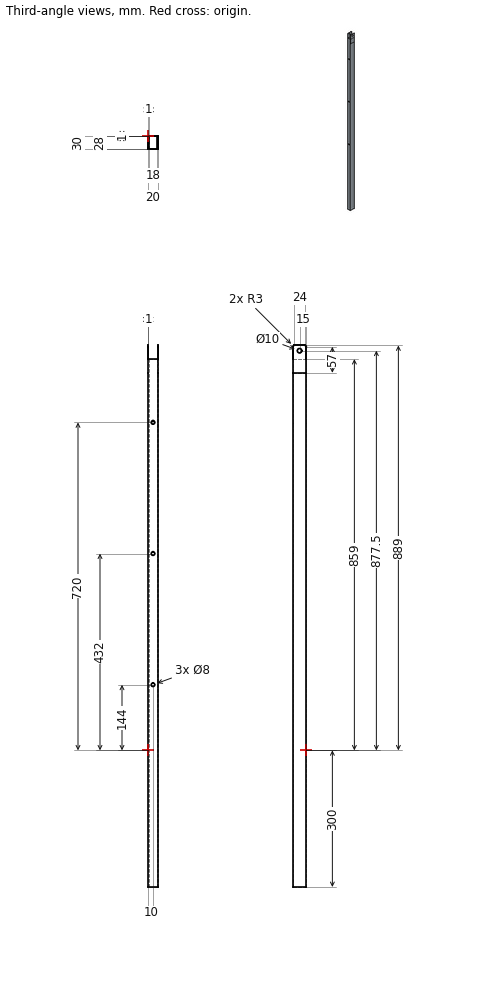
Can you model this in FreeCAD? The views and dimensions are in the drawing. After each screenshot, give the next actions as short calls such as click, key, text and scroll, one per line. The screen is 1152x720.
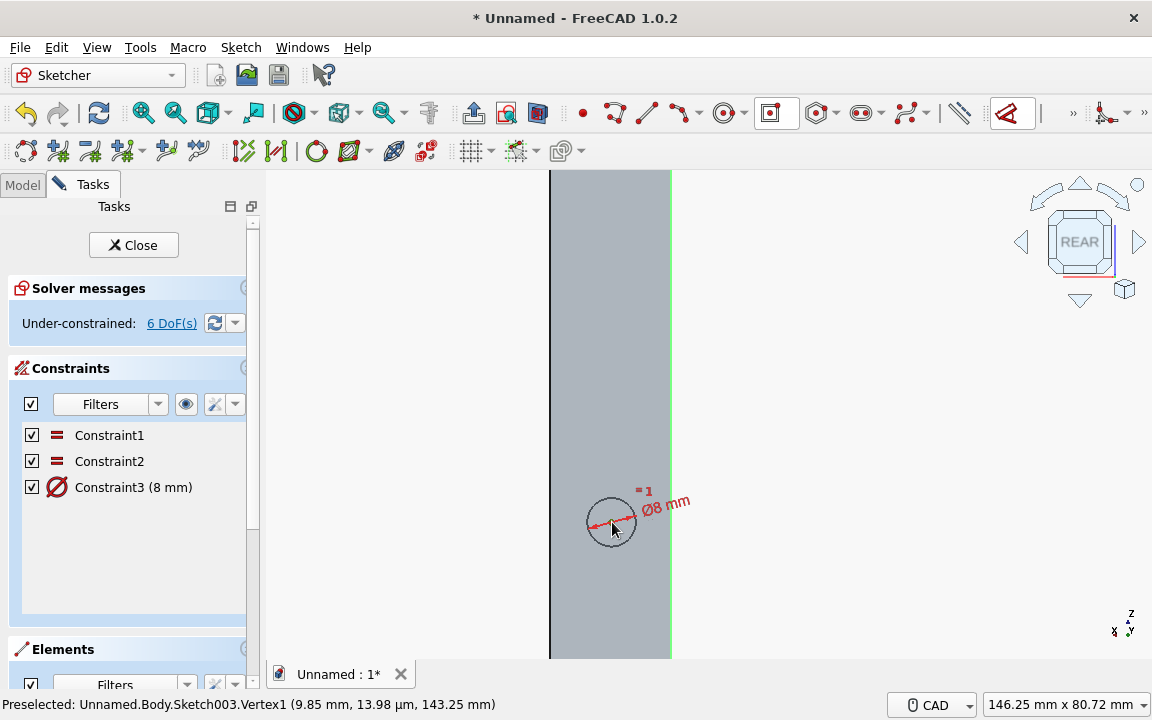
key(l)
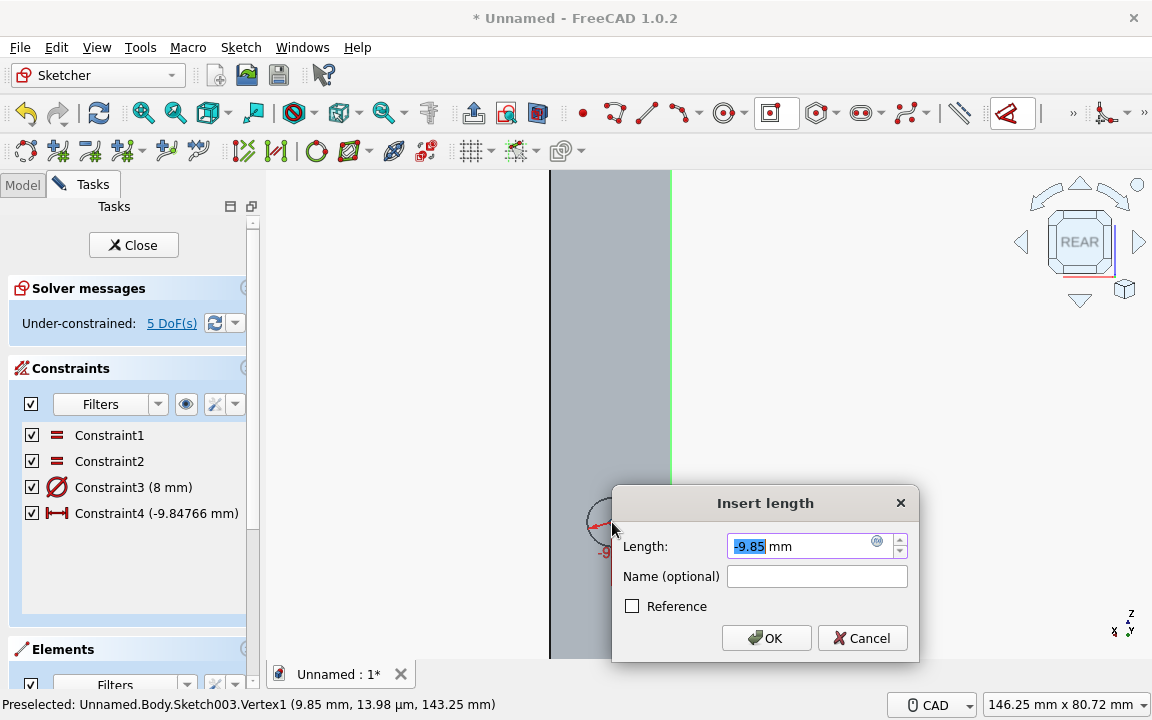
text(-10)
key(Return)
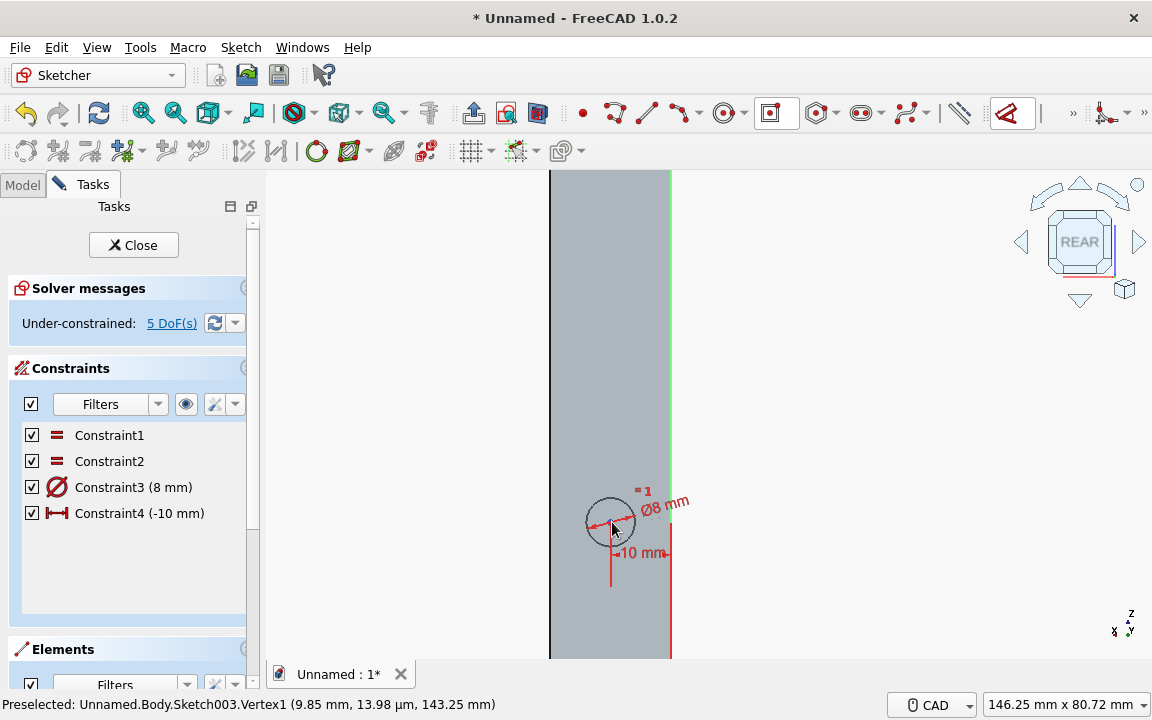
scroll(641, 512, down, 13)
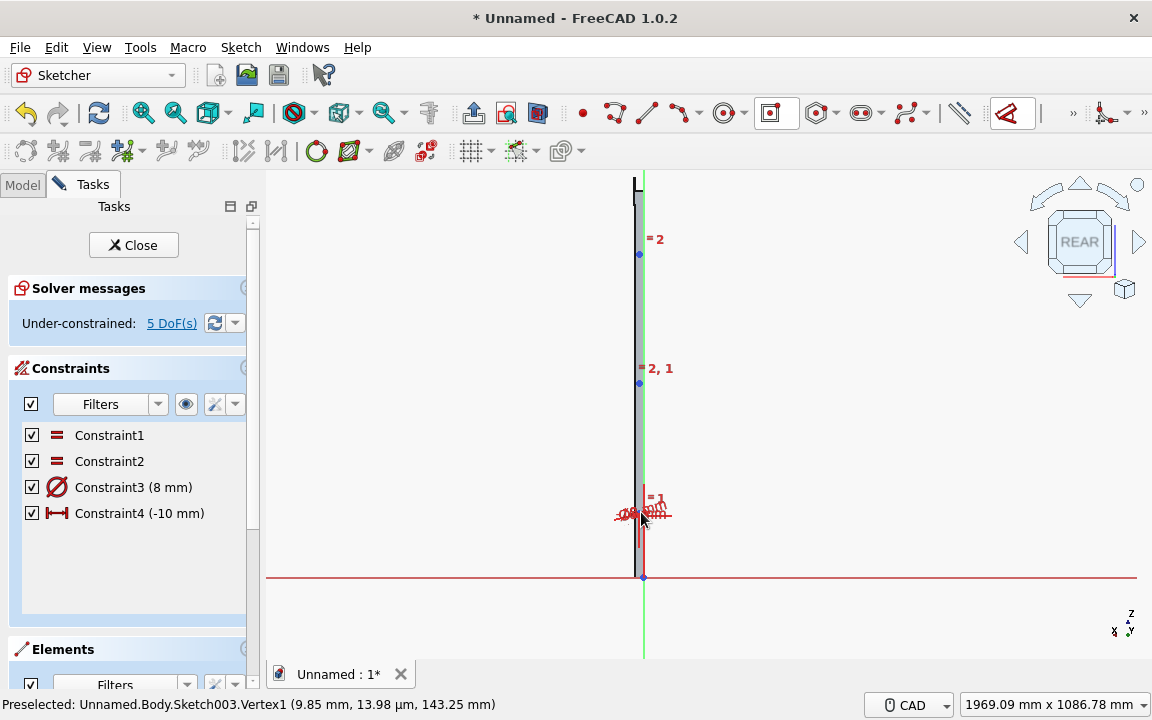
scroll(639, 384, up, 11)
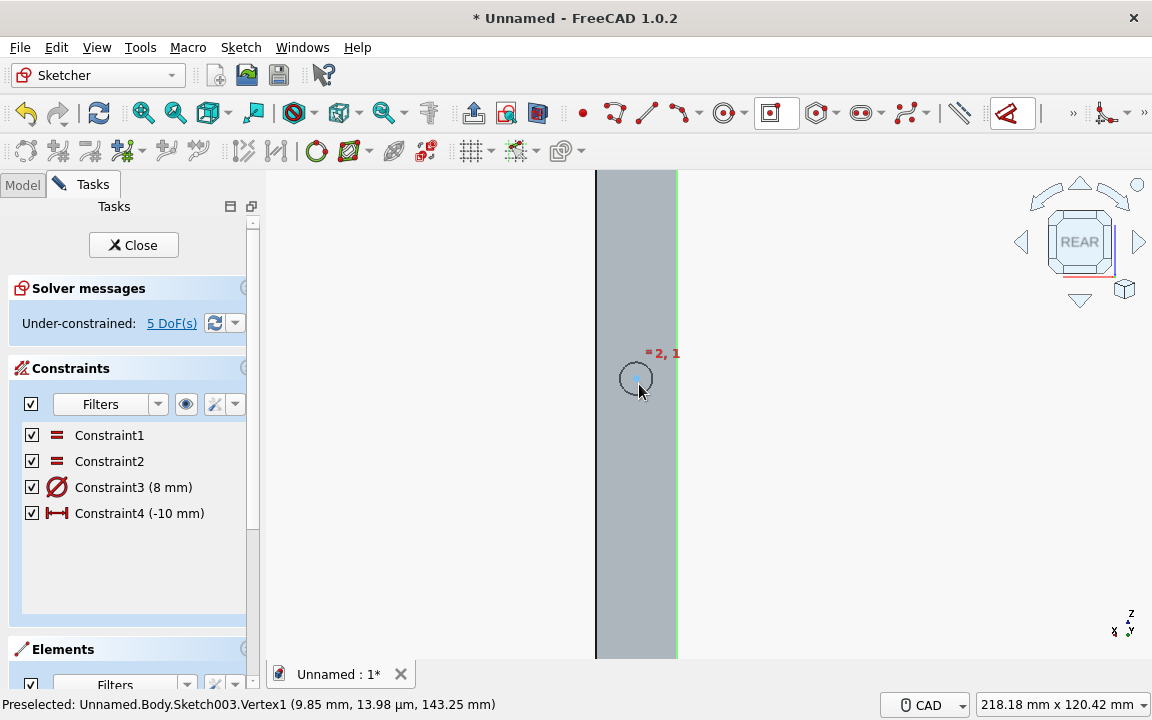
click(636, 379)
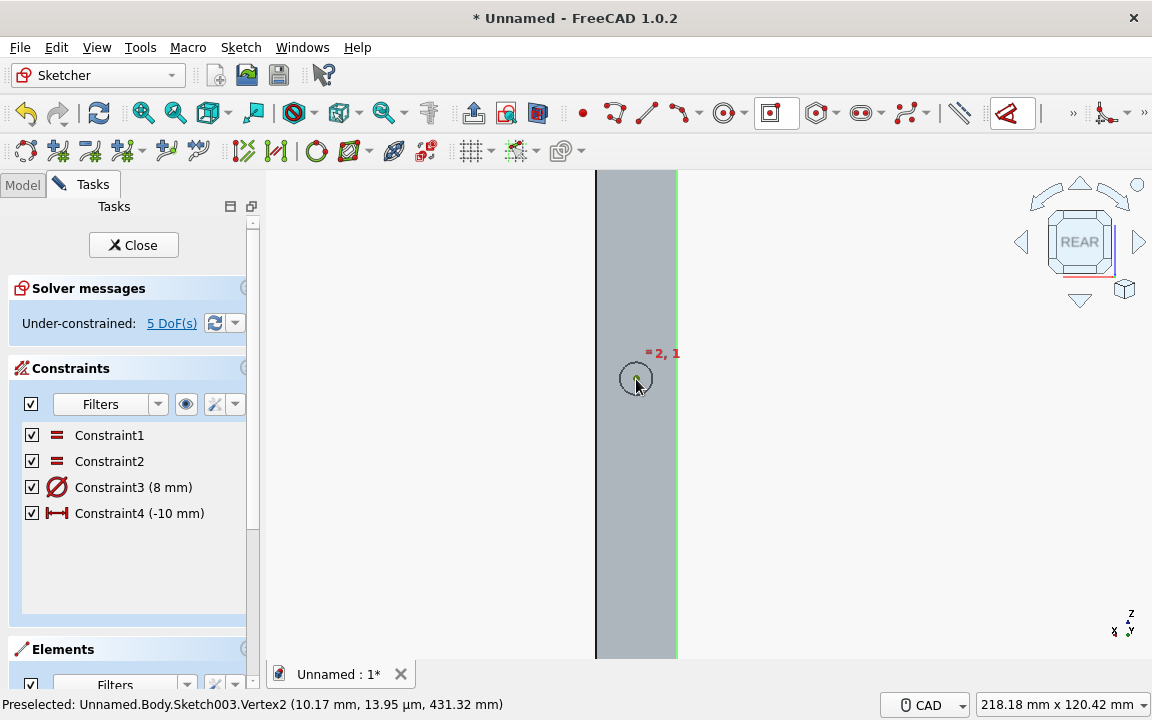
key(l)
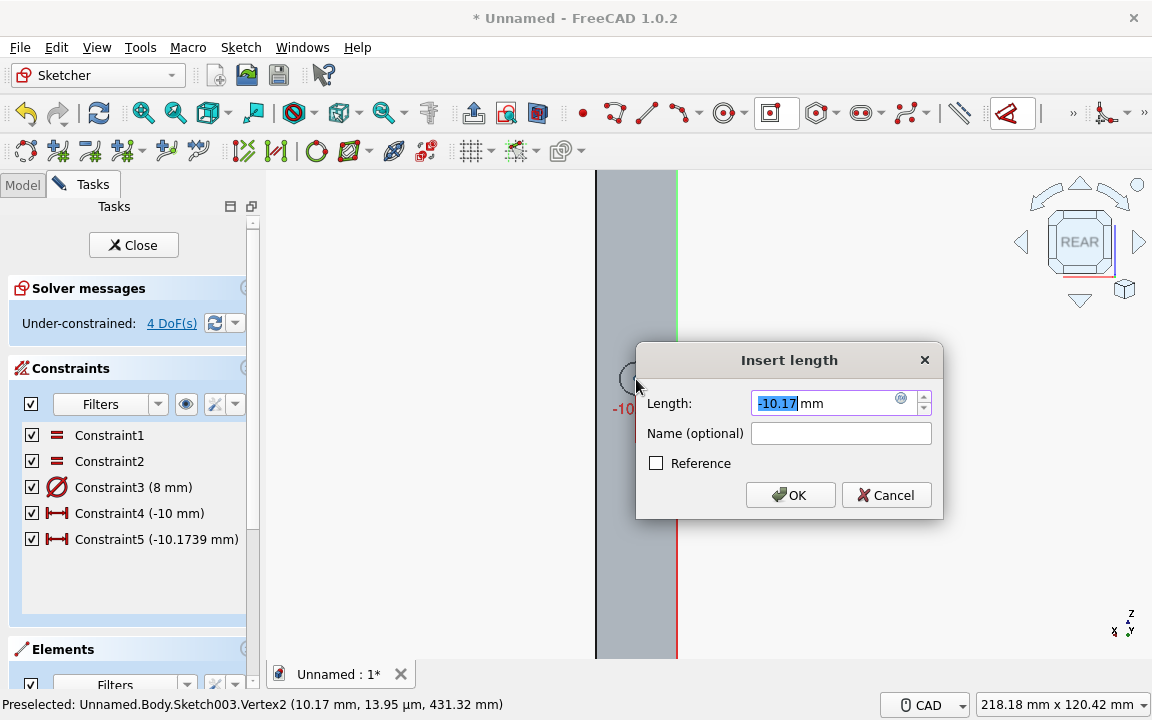
text(-10)
key(Return)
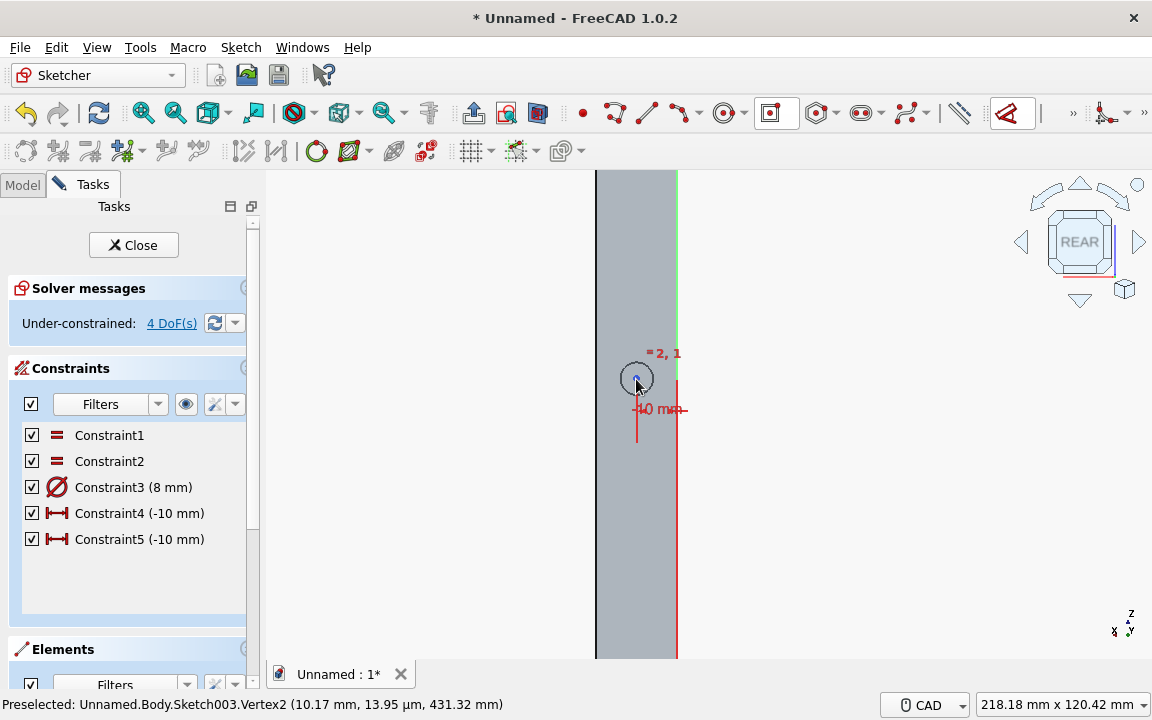
scroll(639, 384, down, 11)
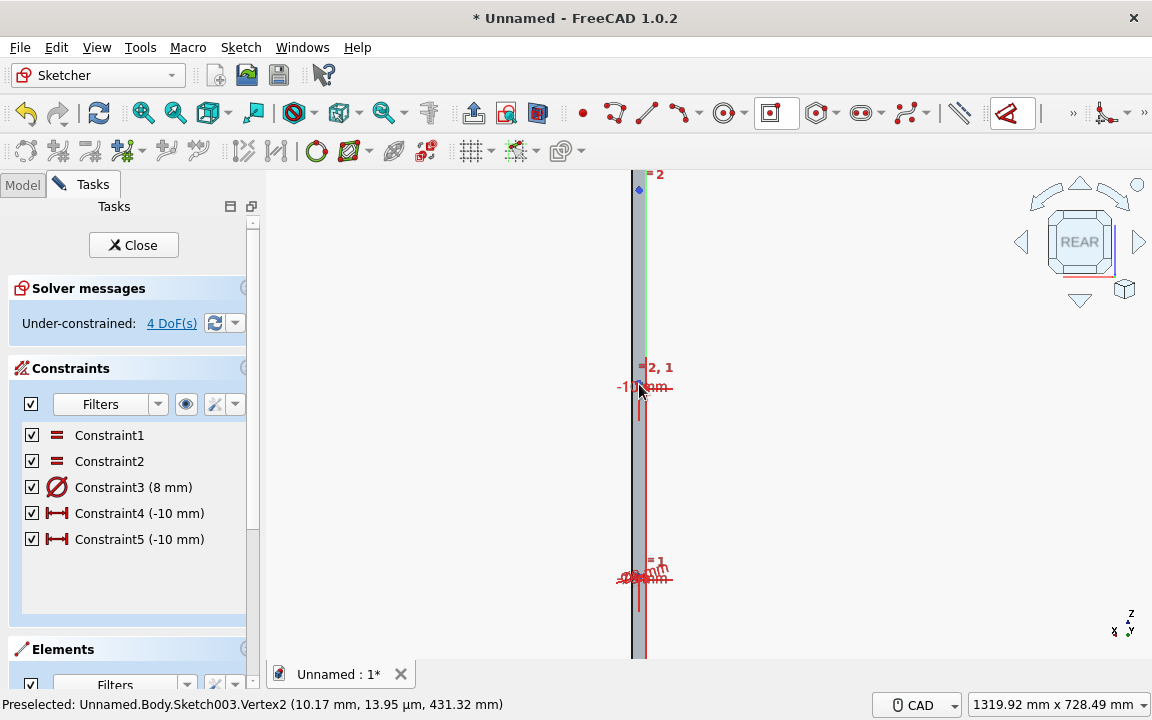
scroll(639, 254, up, 11)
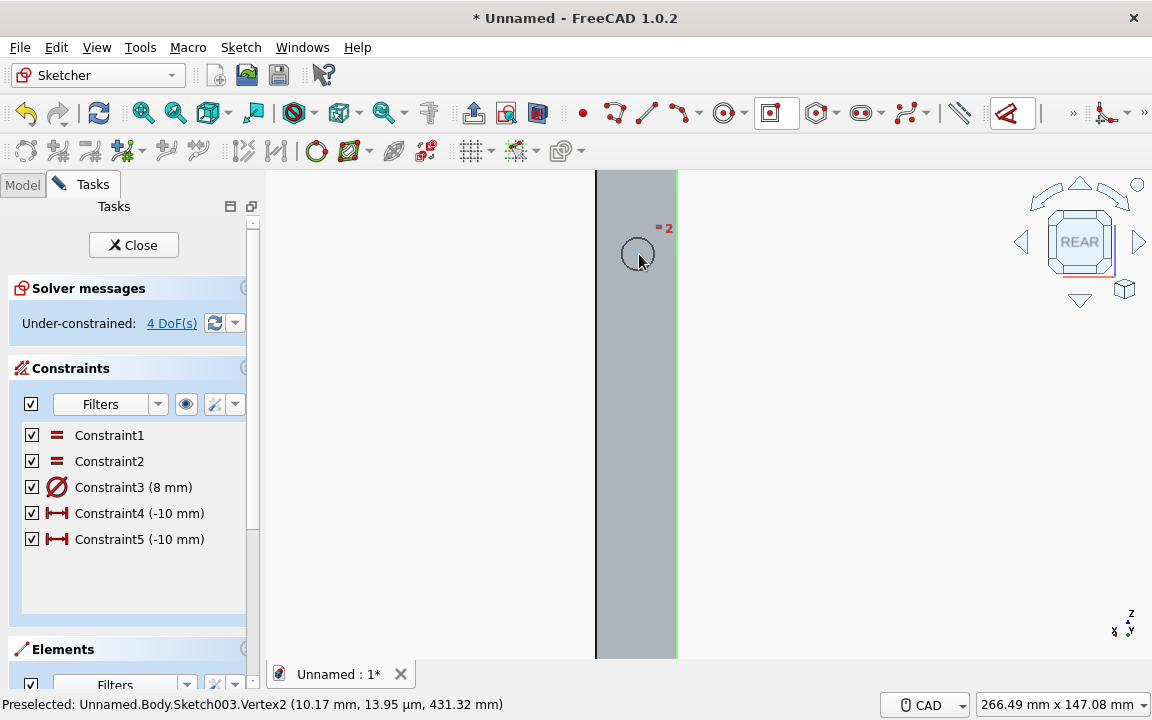
click(638, 254)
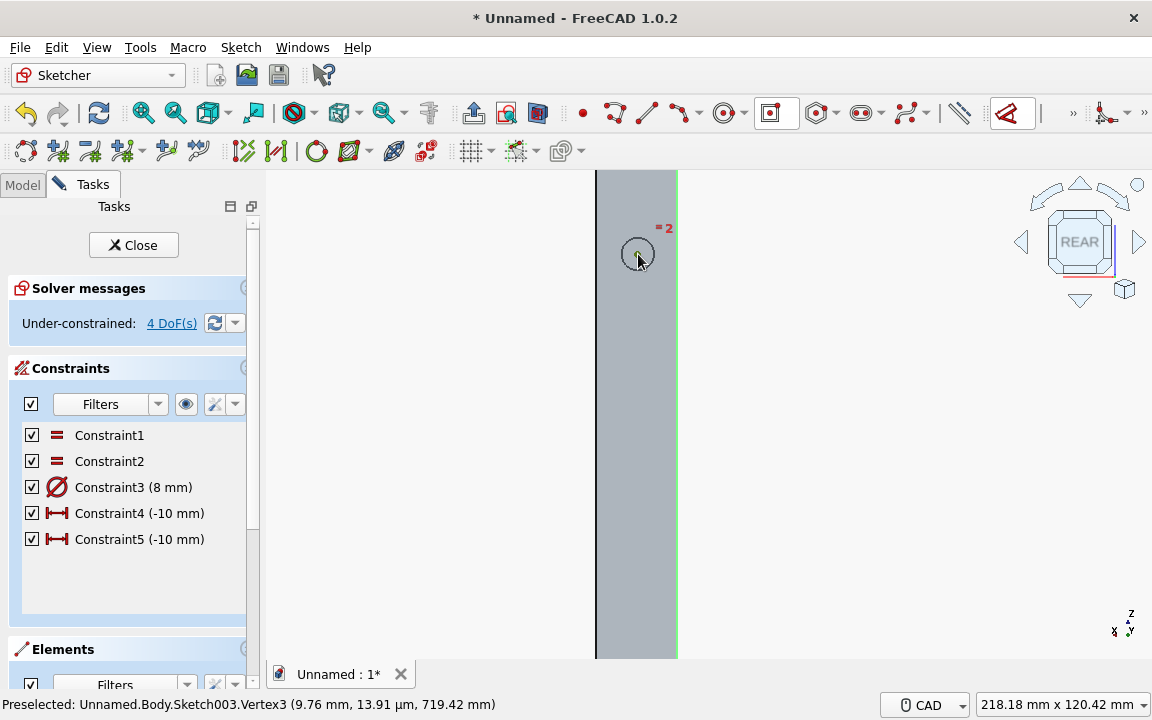
key(l)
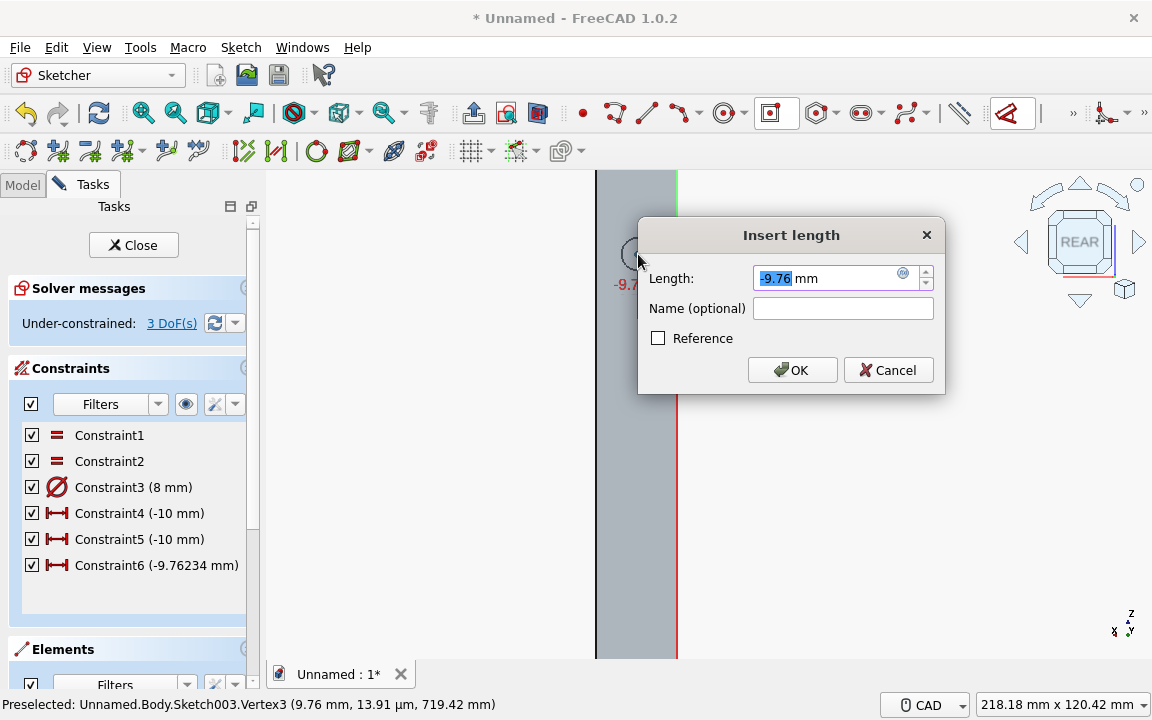
text(-10)
key(Return)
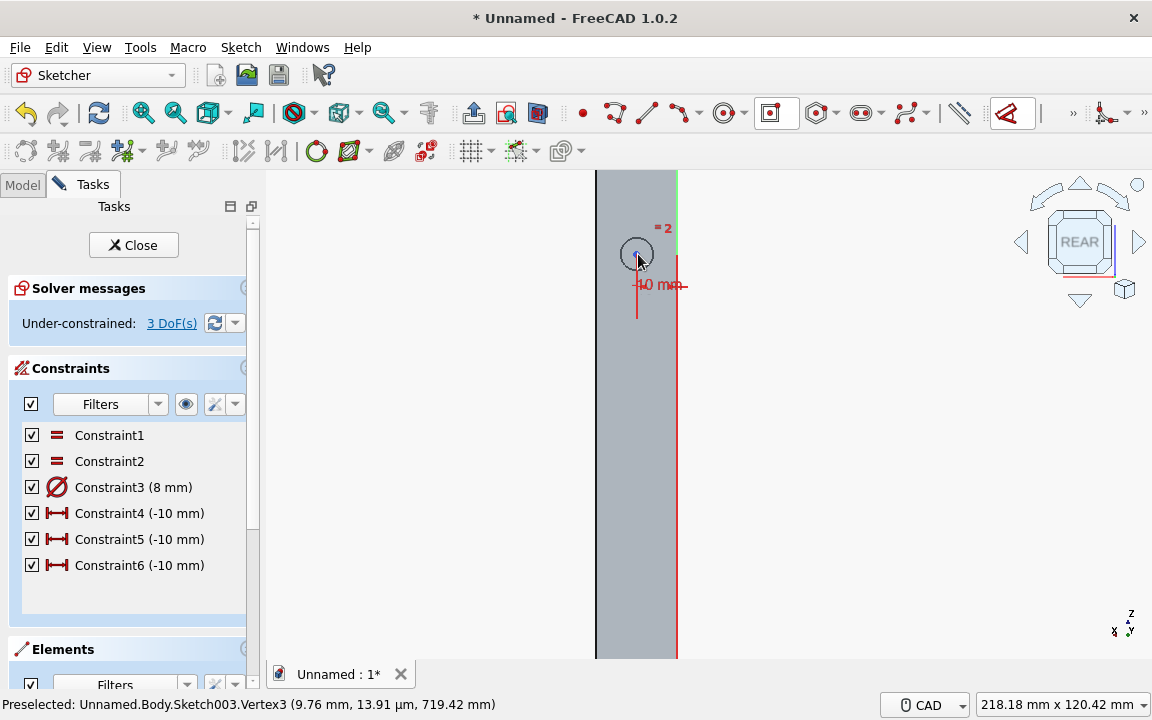
scroll(639, 254, down, 11)